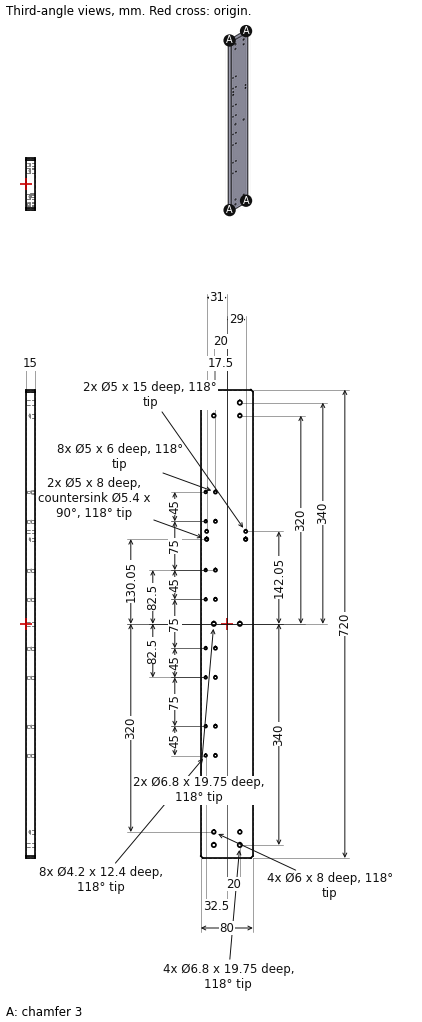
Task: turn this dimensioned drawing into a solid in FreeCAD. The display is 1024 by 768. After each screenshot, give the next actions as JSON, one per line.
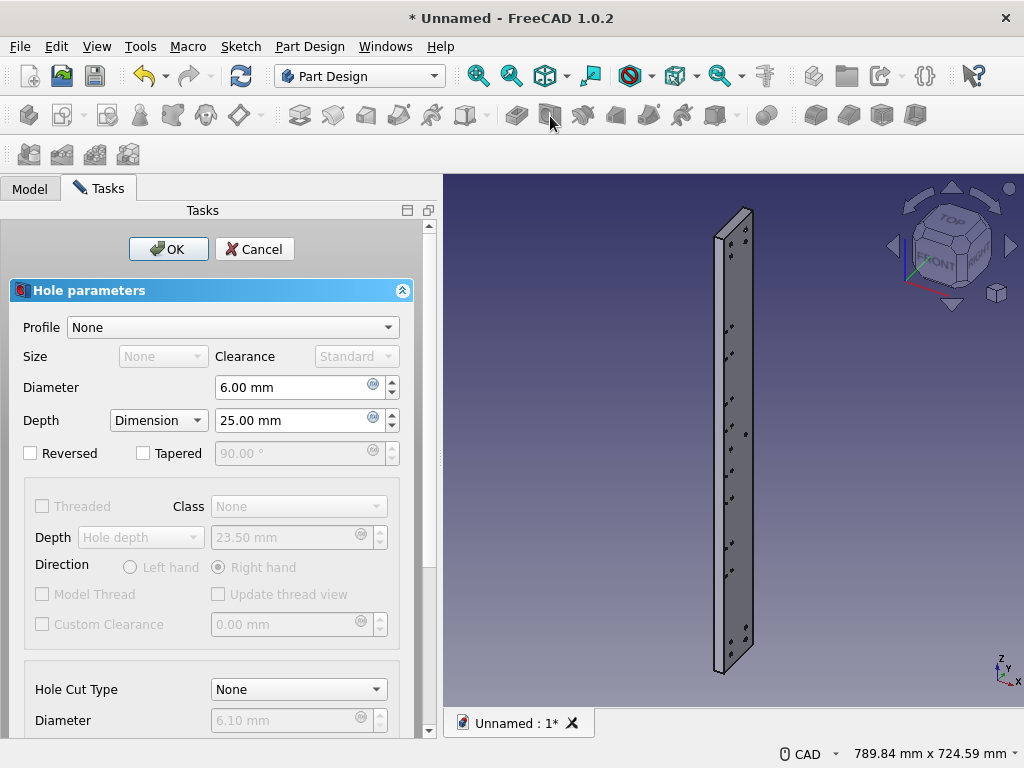
{"action": "triple_click", "coordinate": [300, 388]}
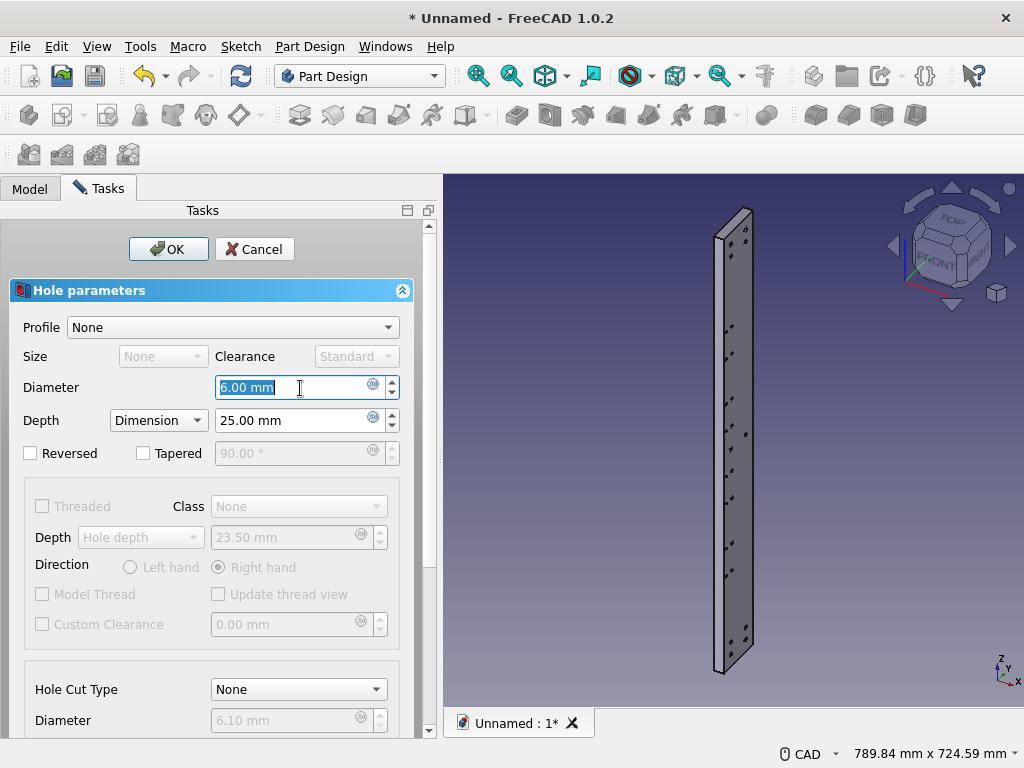
{"action": "type", "text": "6.8"}
{"action": "key", "text": "Tab"}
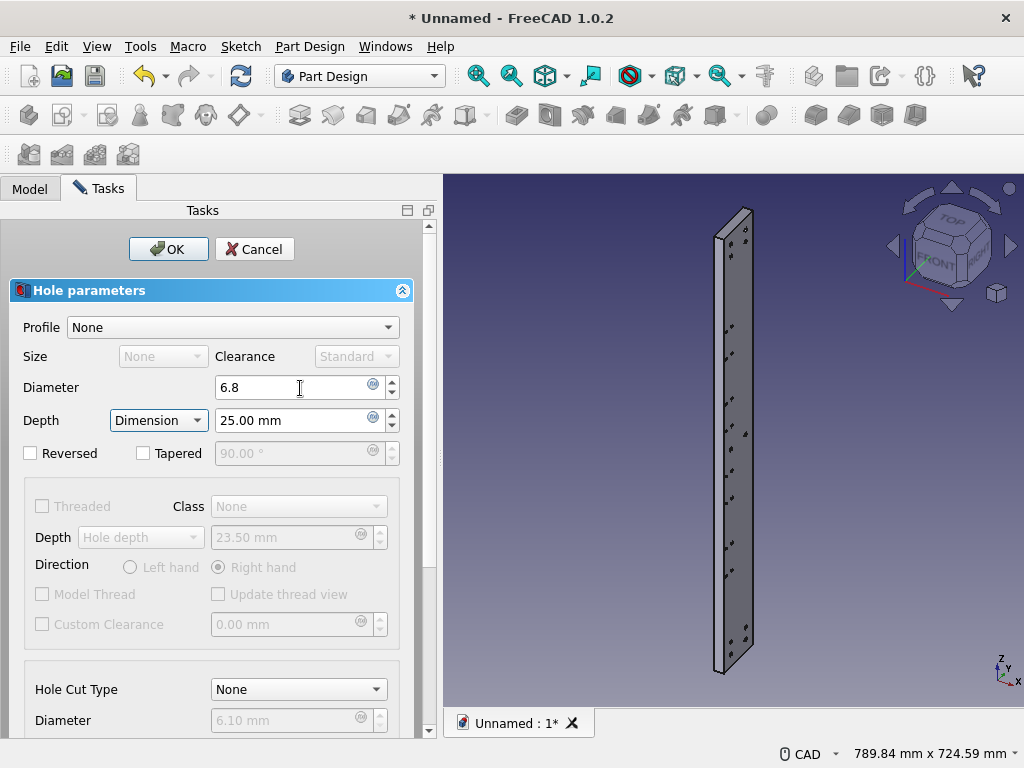
{"action": "triple_click", "coordinate": [300, 420]}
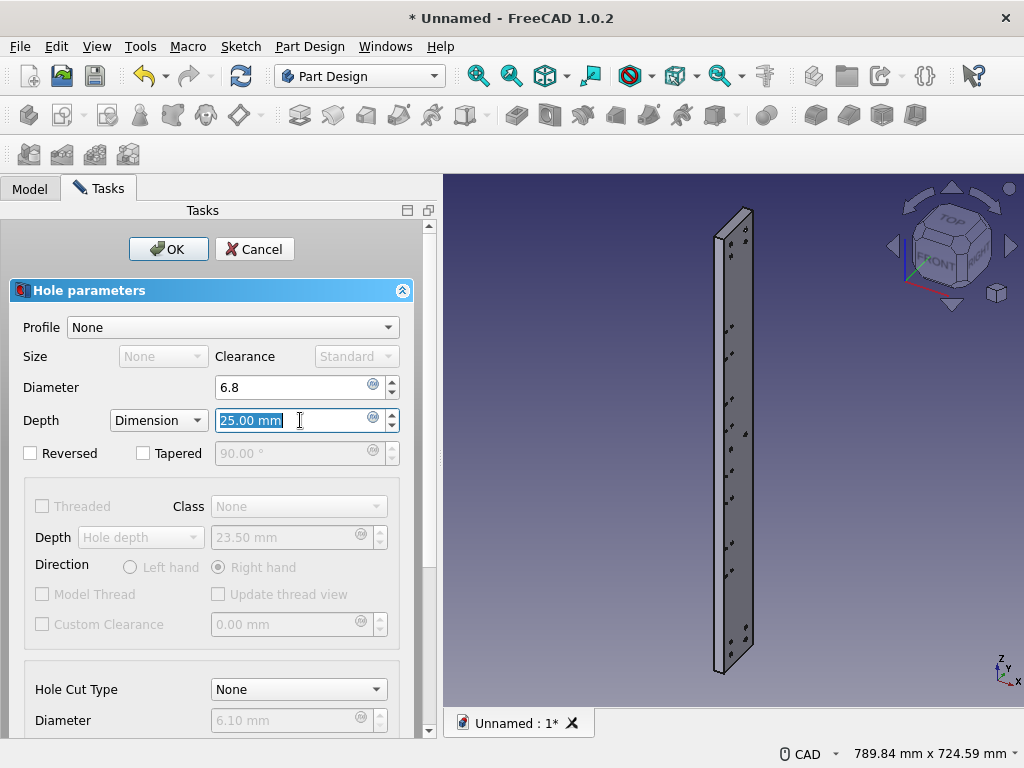
{"action": "type", "text": "19.75"}
{"action": "key", "text": "Tab"}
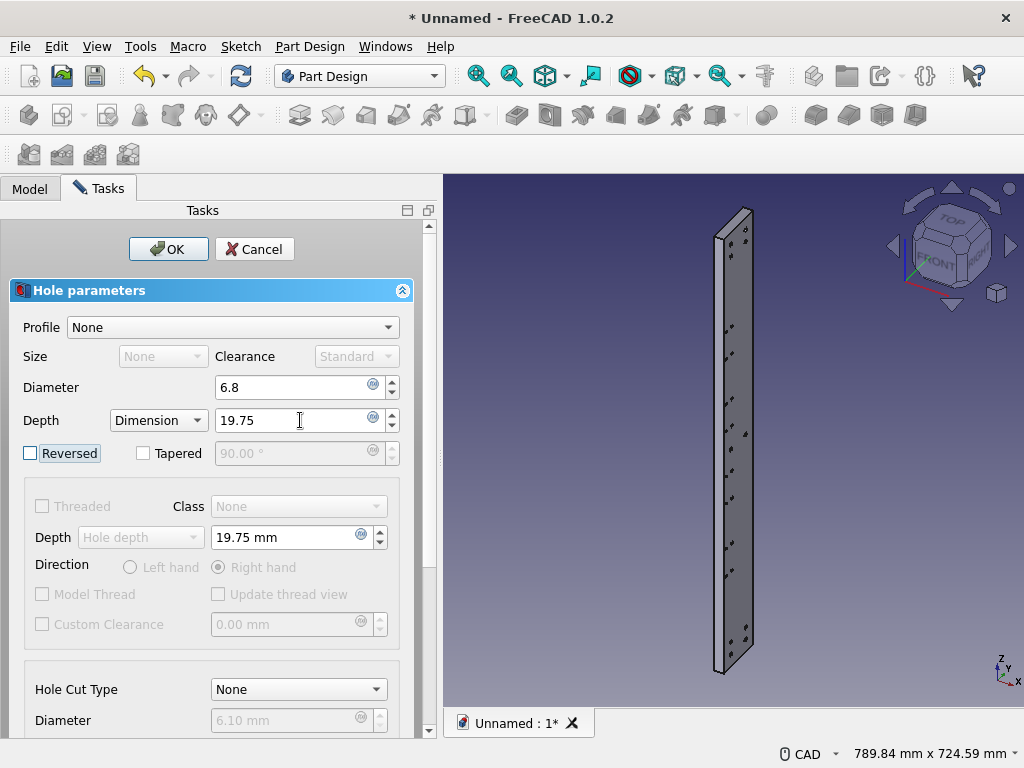
{"action": "left_click", "coordinate": [169, 249]}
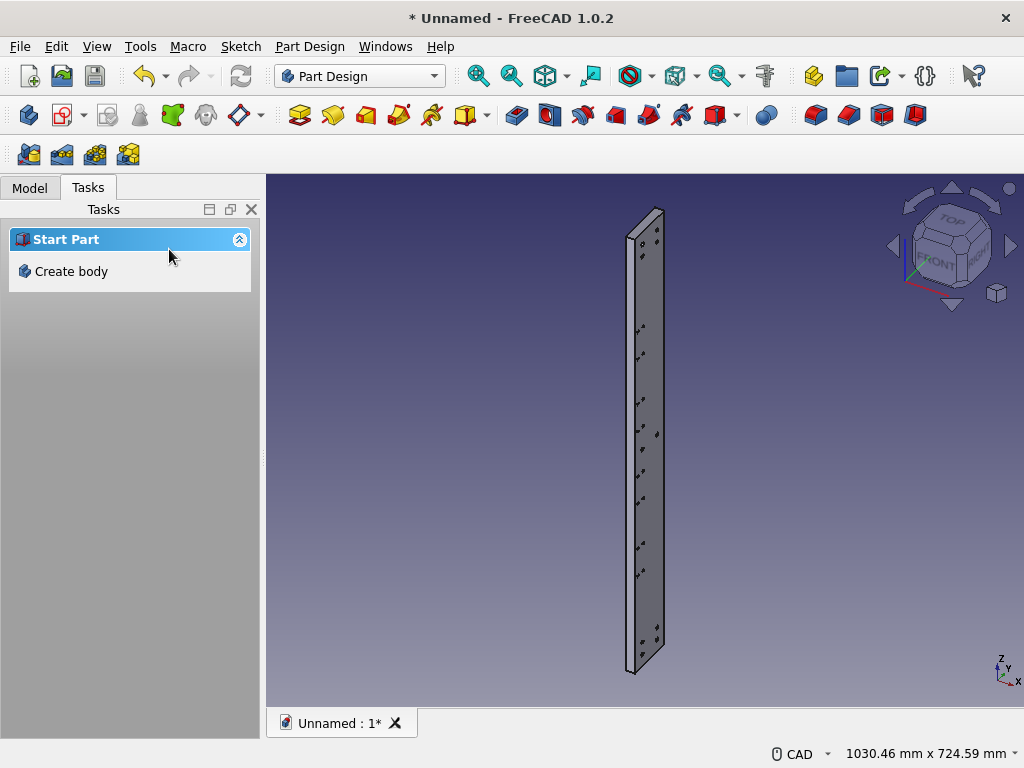
{"action": "left_click", "coordinate": [654, 499]}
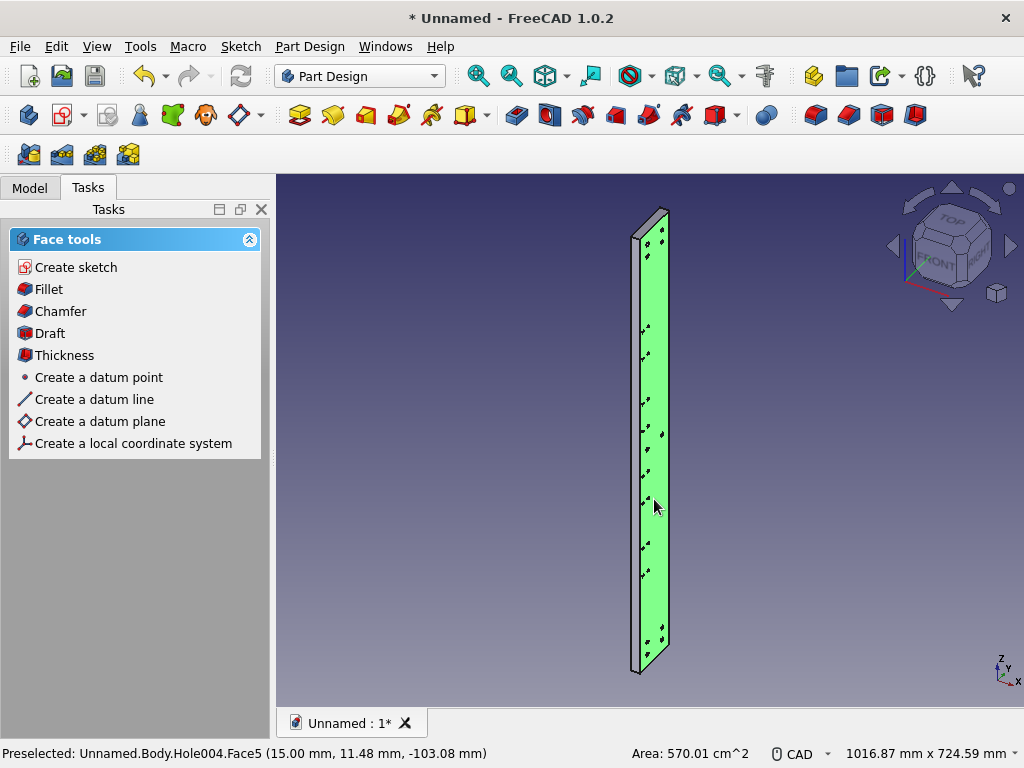
{"action": "left_click", "coordinate": [62, 116]}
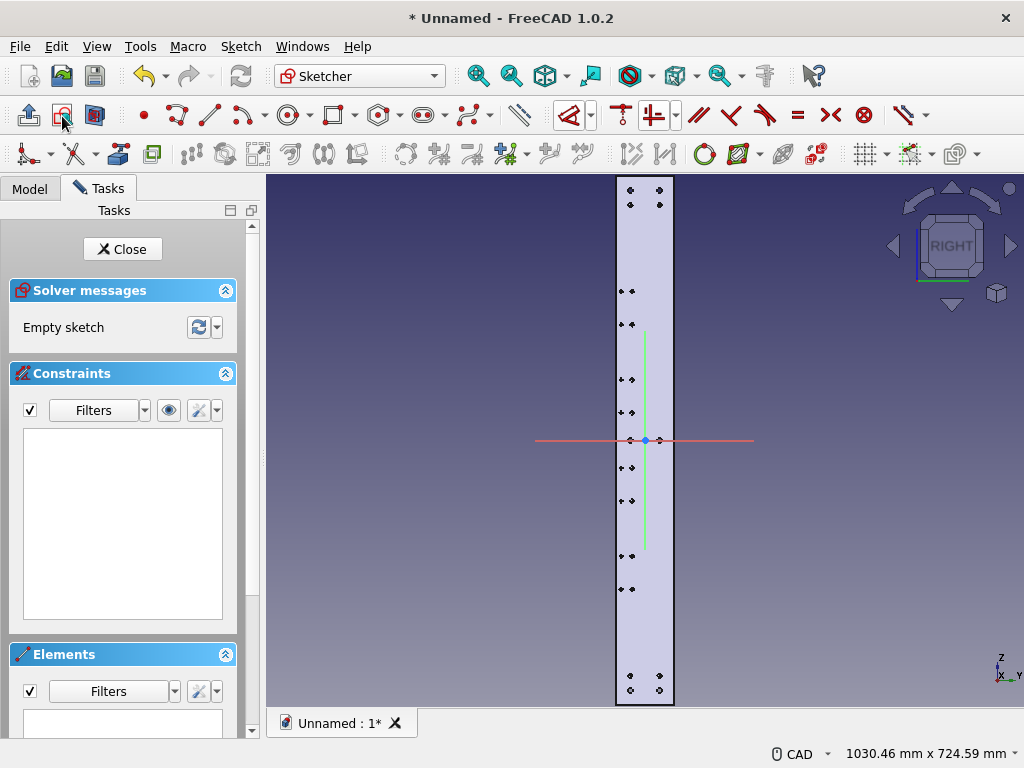
{"action": "scroll", "coordinate": [673, 364], "scroll_direction": "up", "scroll_amount": 6}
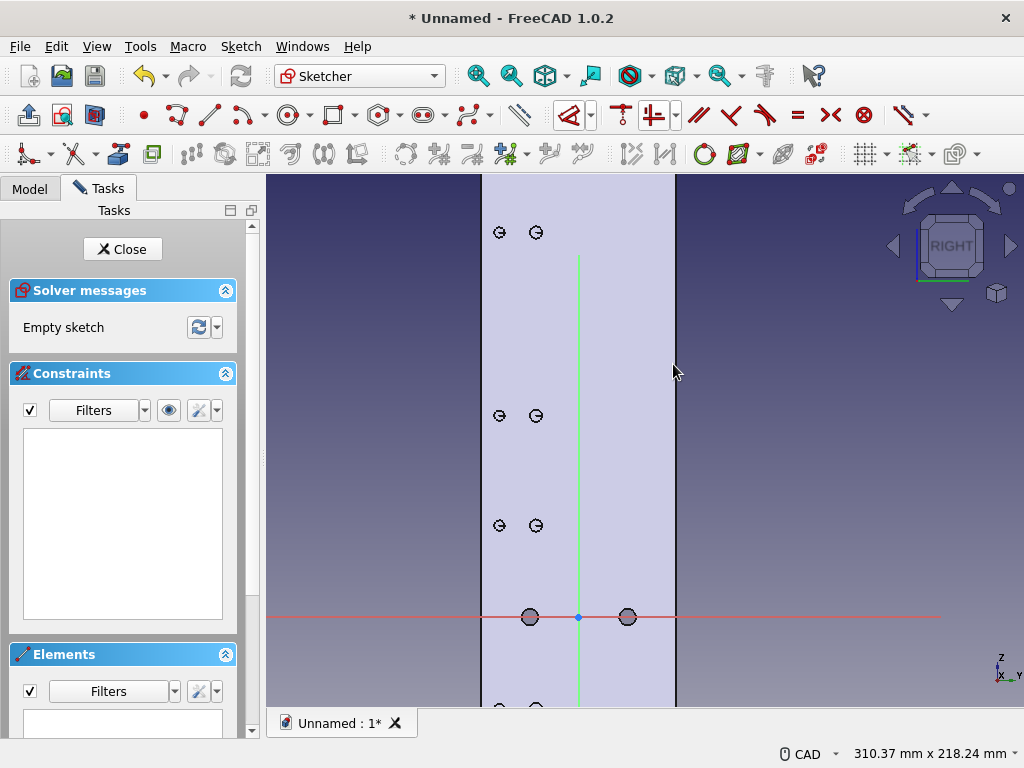
{"action": "left_click", "coordinate": [288, 116]}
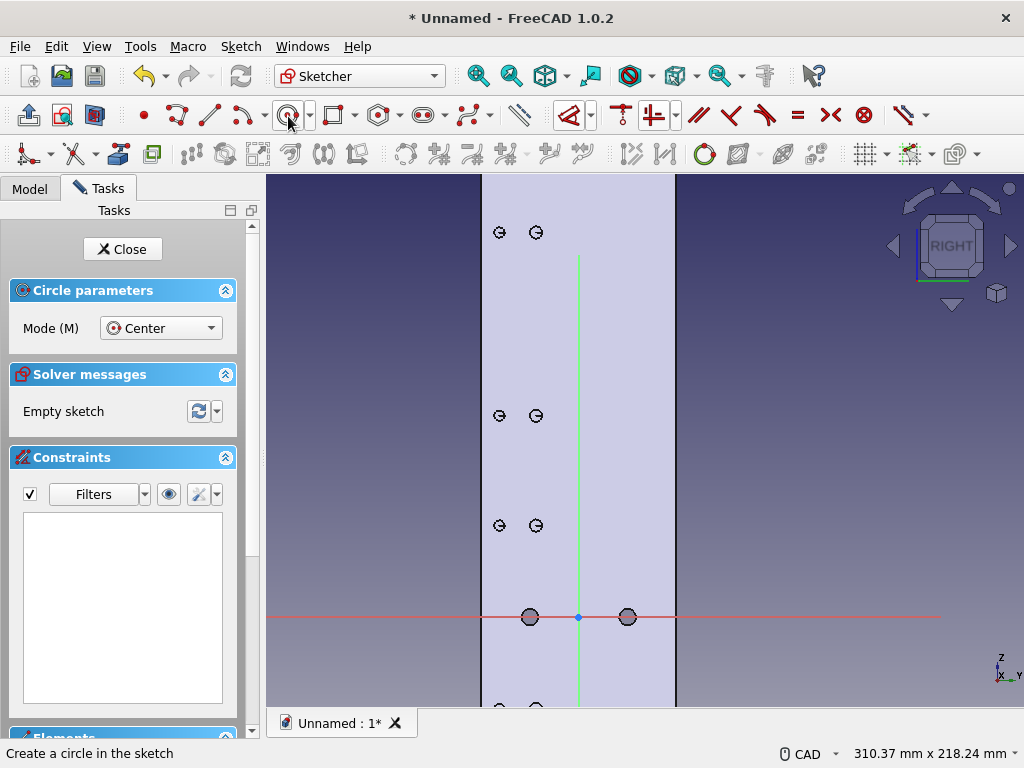
{"action": "scroll", "coordinate": [650, 270], "scroll_direction": "up", "scroll_amount": 7}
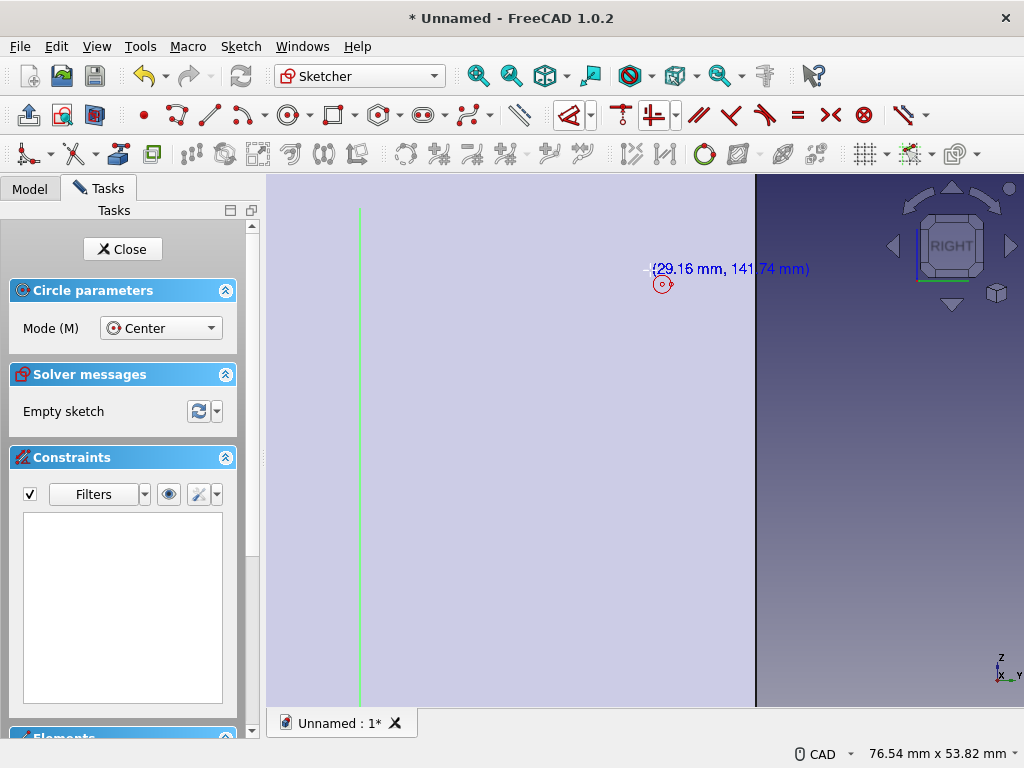
{"action": "scroll", "coordinate": [651, 270], "scroll_direction": "down", "scroll_amount": 7}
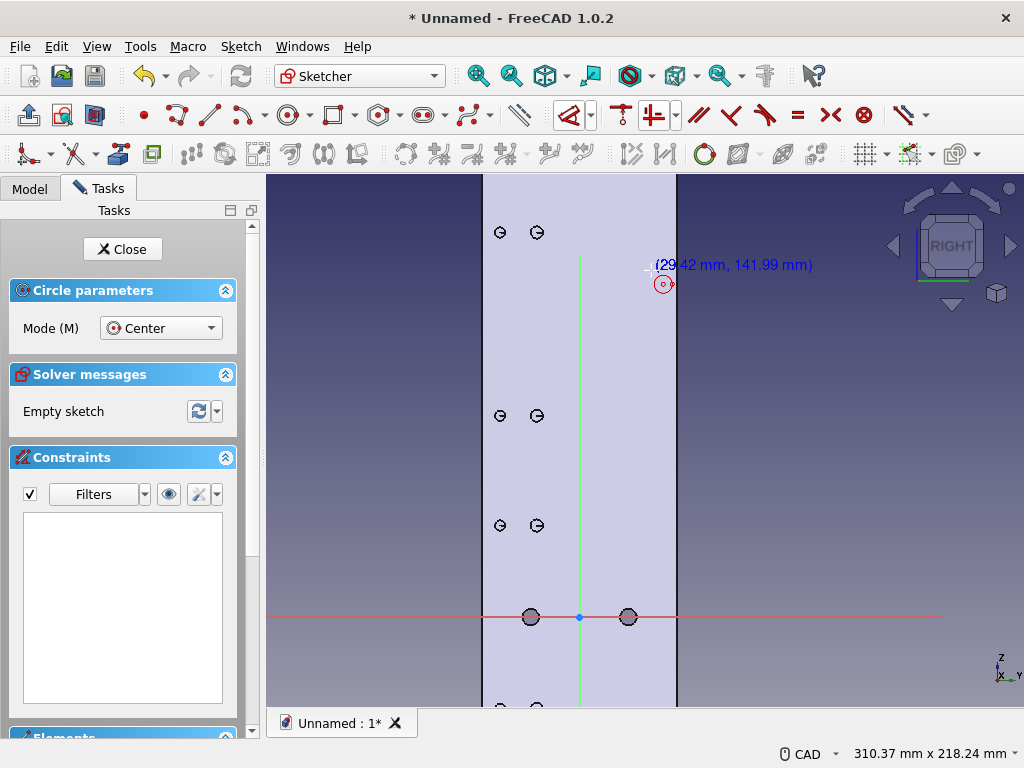
{"action": "left_click", "coordinate": [650, 270]}
{"action": "mouse_move", "coordinate": [655, 266]}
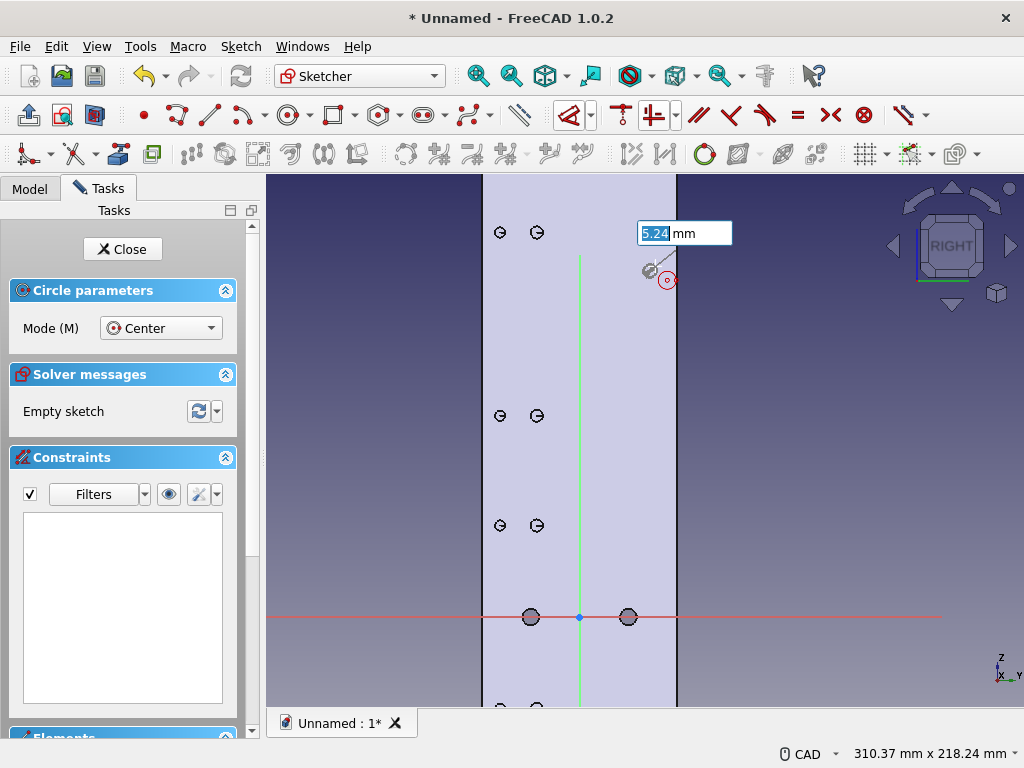
{"action": "type", "text": "5"}
{"action": "key", "text": "Return"}